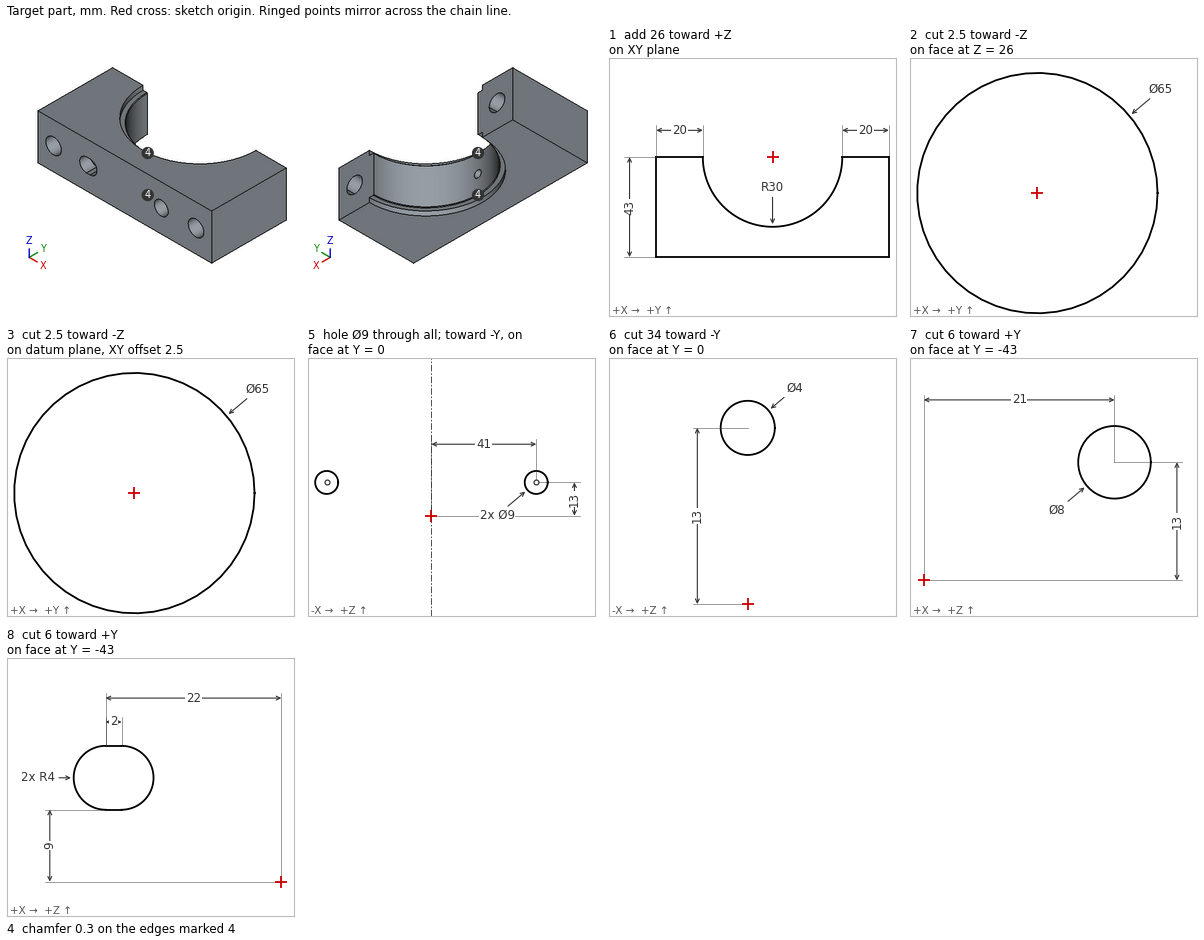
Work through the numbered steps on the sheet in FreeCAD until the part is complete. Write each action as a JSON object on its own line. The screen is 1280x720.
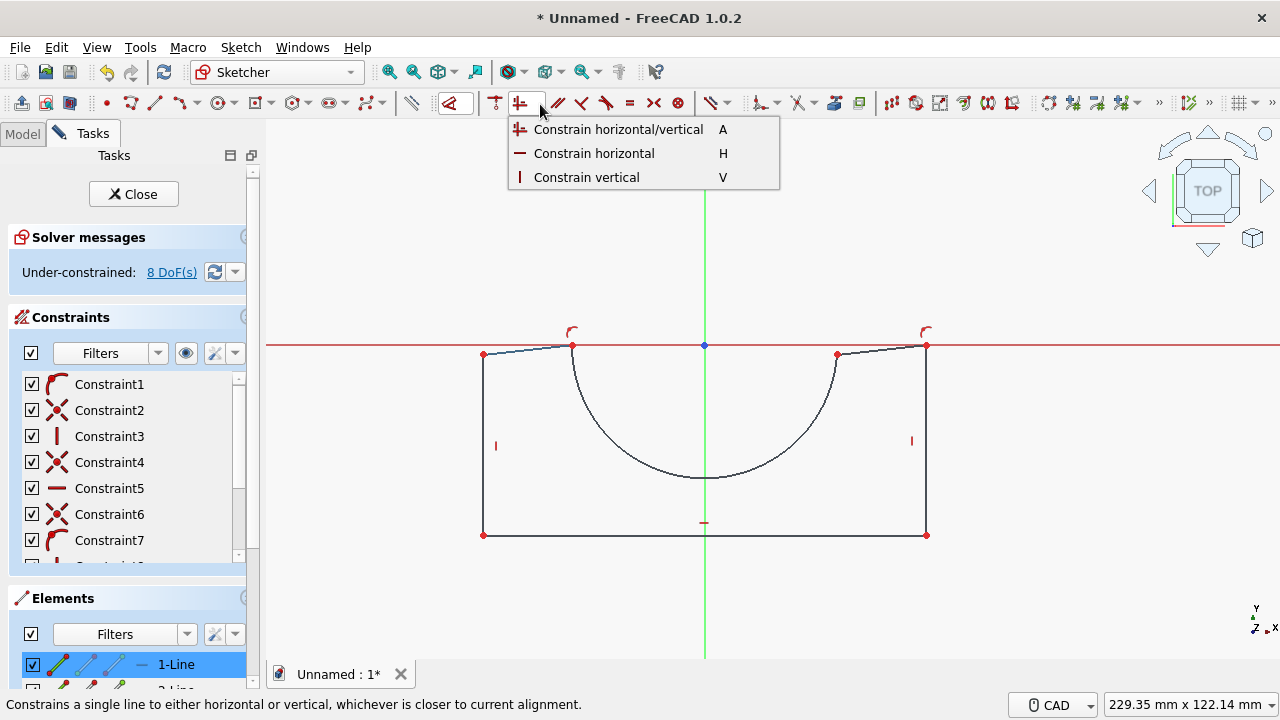
{"action": "left_click", "coordinate": [644, 153]}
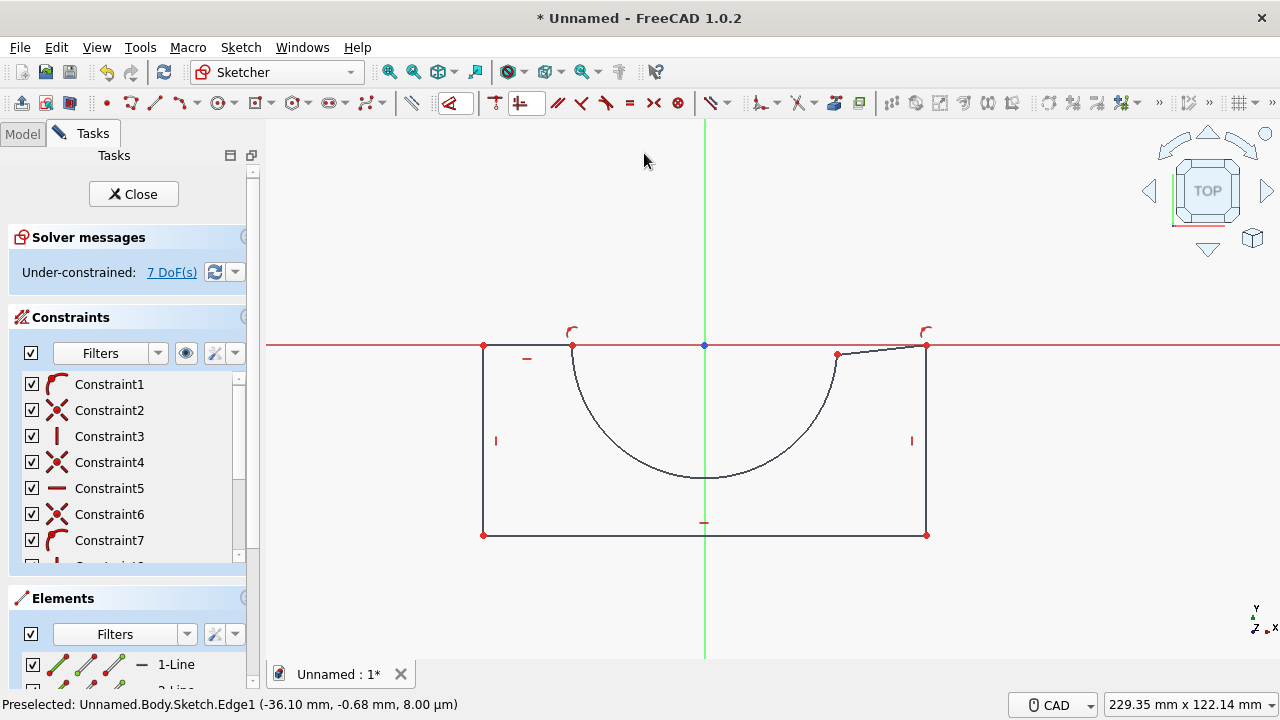
{"action": "left_click", "coordinate": [899, 348]}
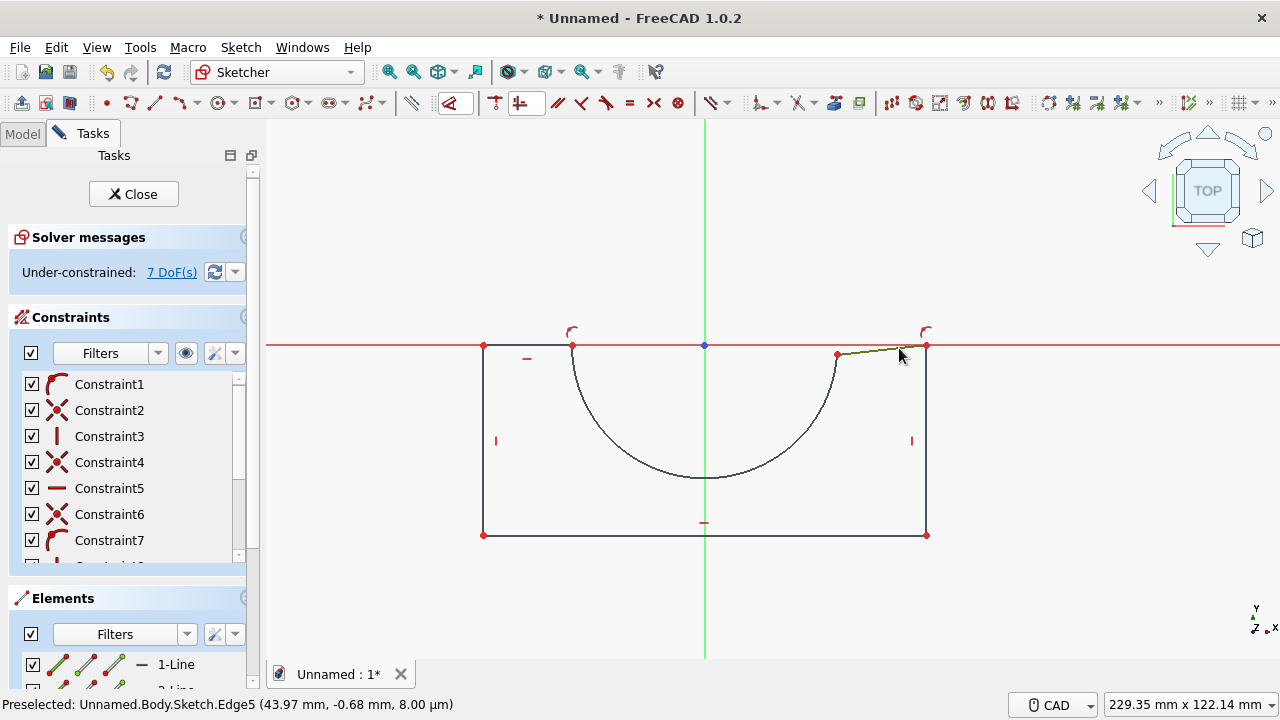
{"action": "key", "text": "h"}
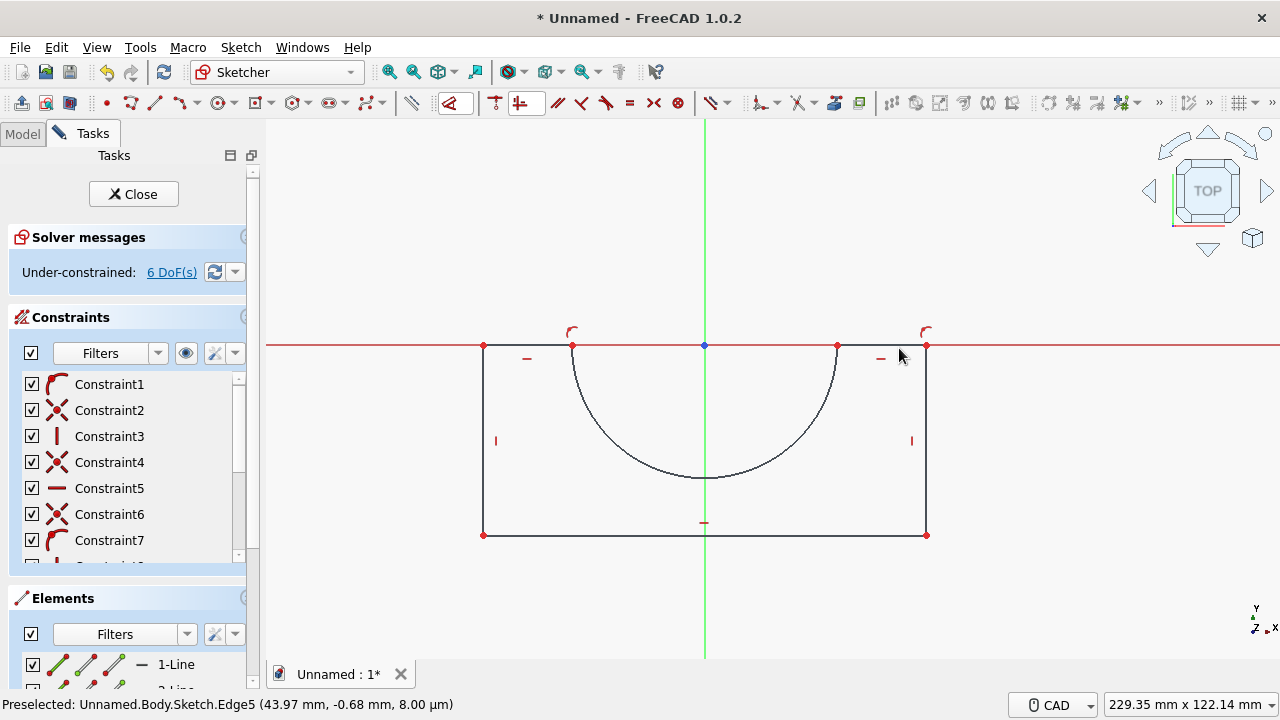
{"action": "left_click_drag", "start_coordinate": [695, 335], "coordinate": [715, 356]}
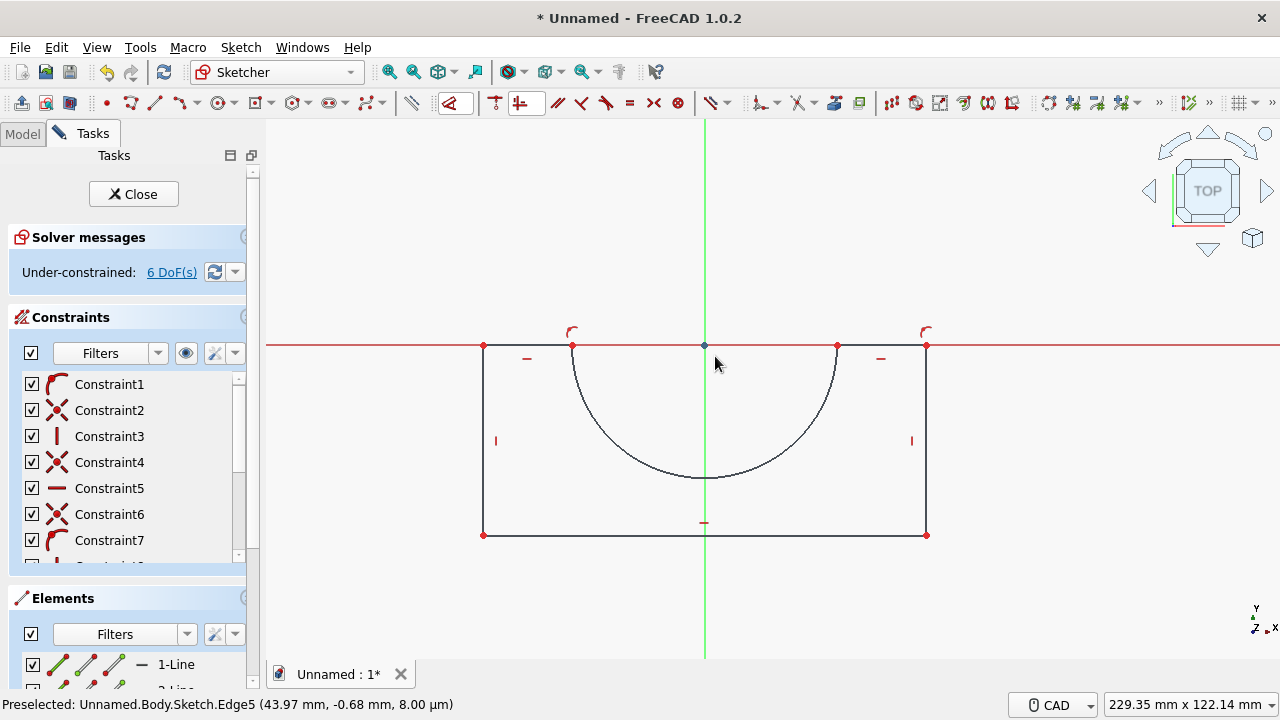
{"action": "left_click", "coordinate": [496, 104]}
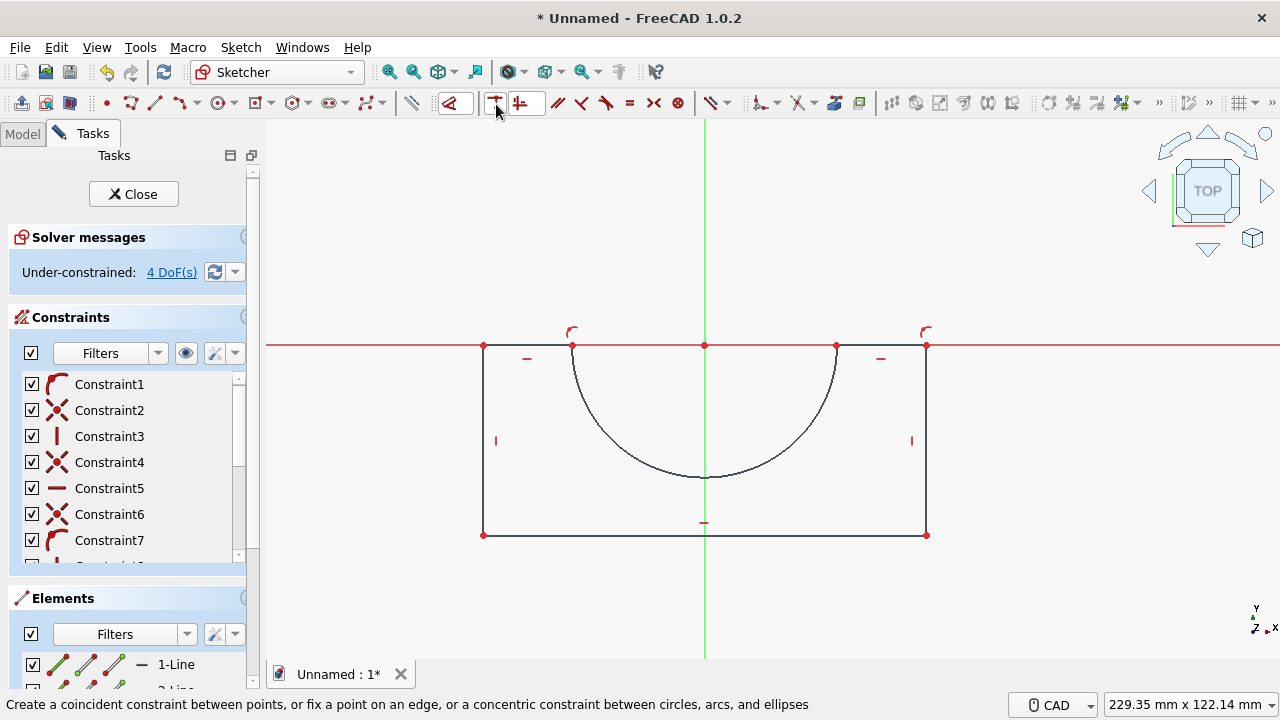
{"action": "left_click", "coordinate": [627, 452]}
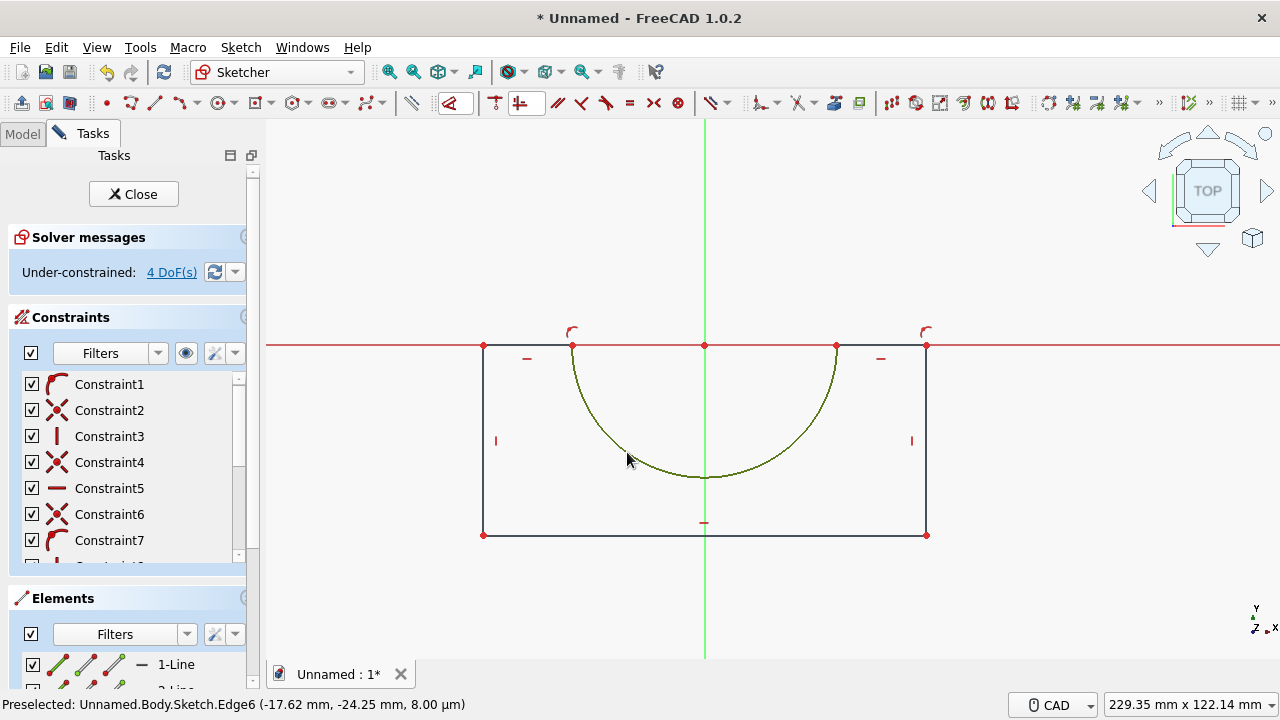
{"action": "left_click", "coordinate": [468, 104]}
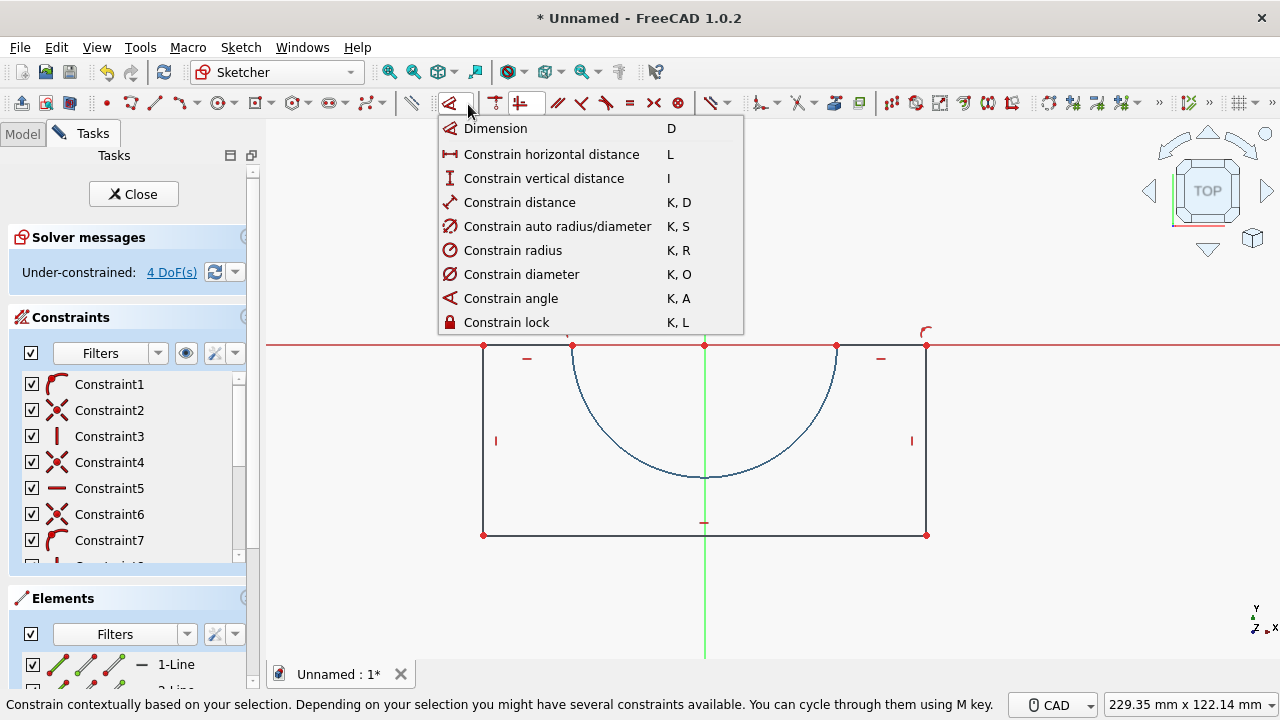
{"action": "left_click", "coordinate": [591, 250]}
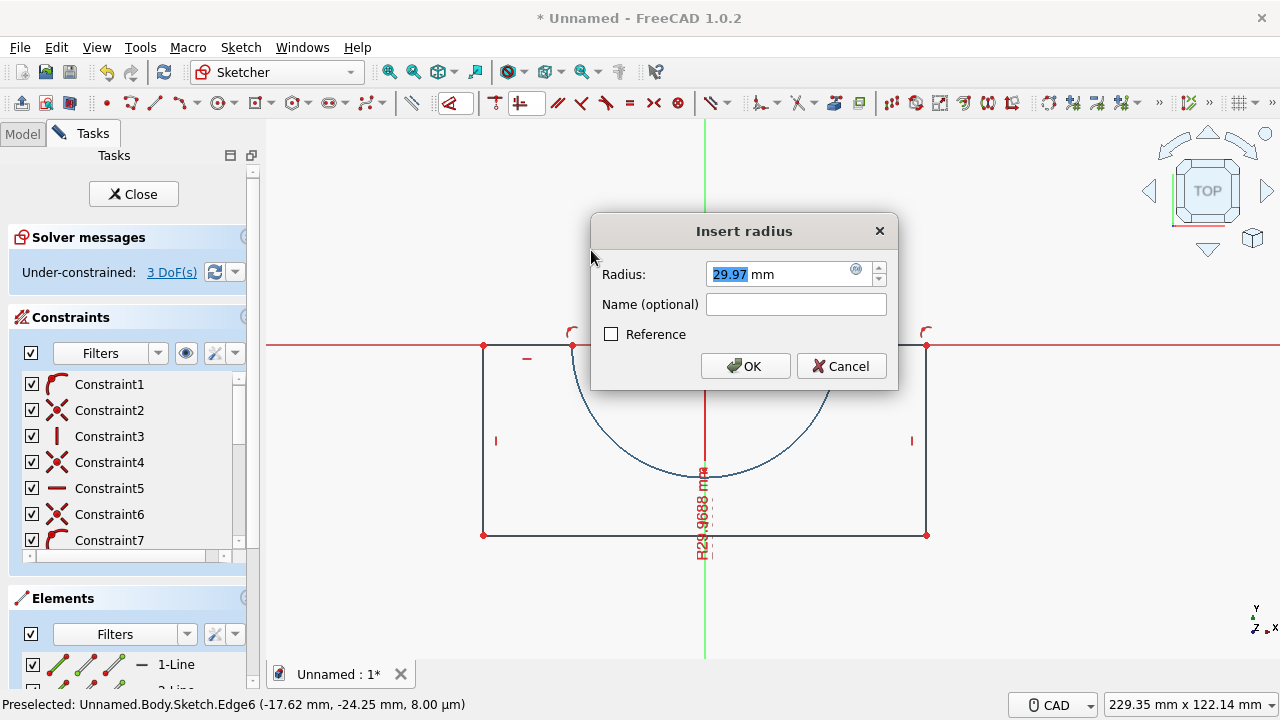
{"action": "type", "text": "30"}
{"action": "key", "text": "Return"}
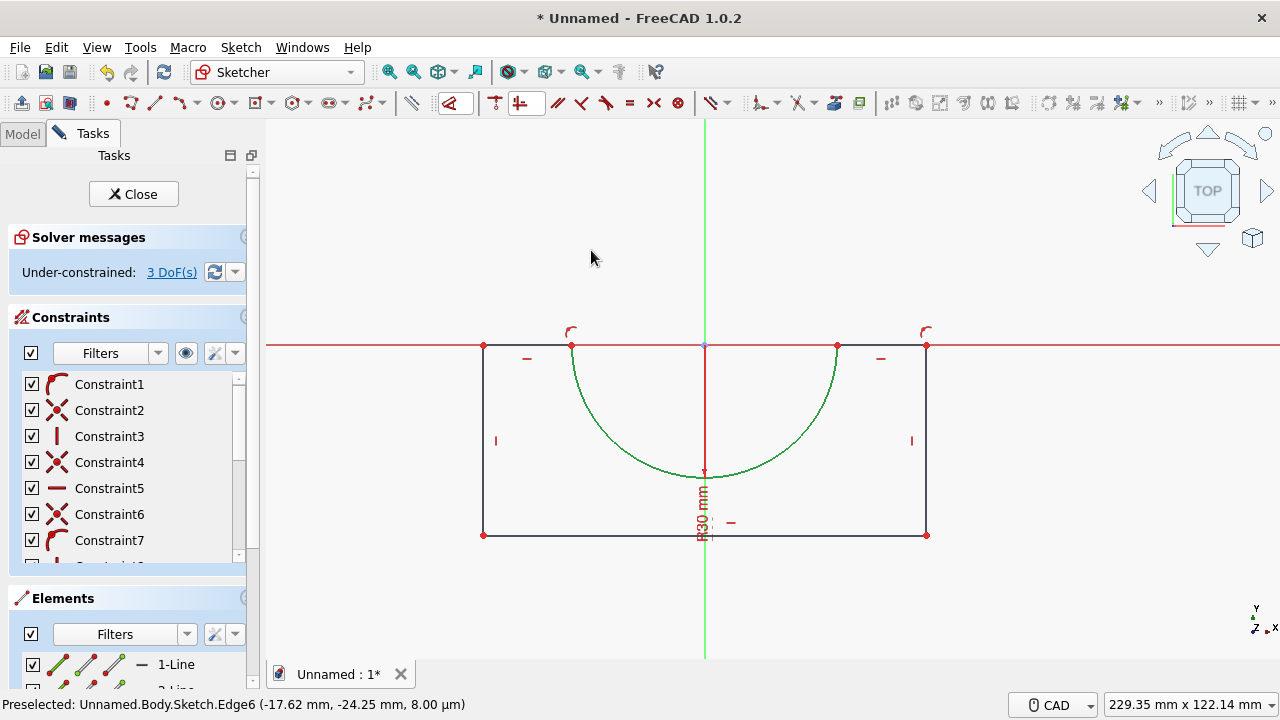
{"action": "left_click", "coordinate": [545, 345]}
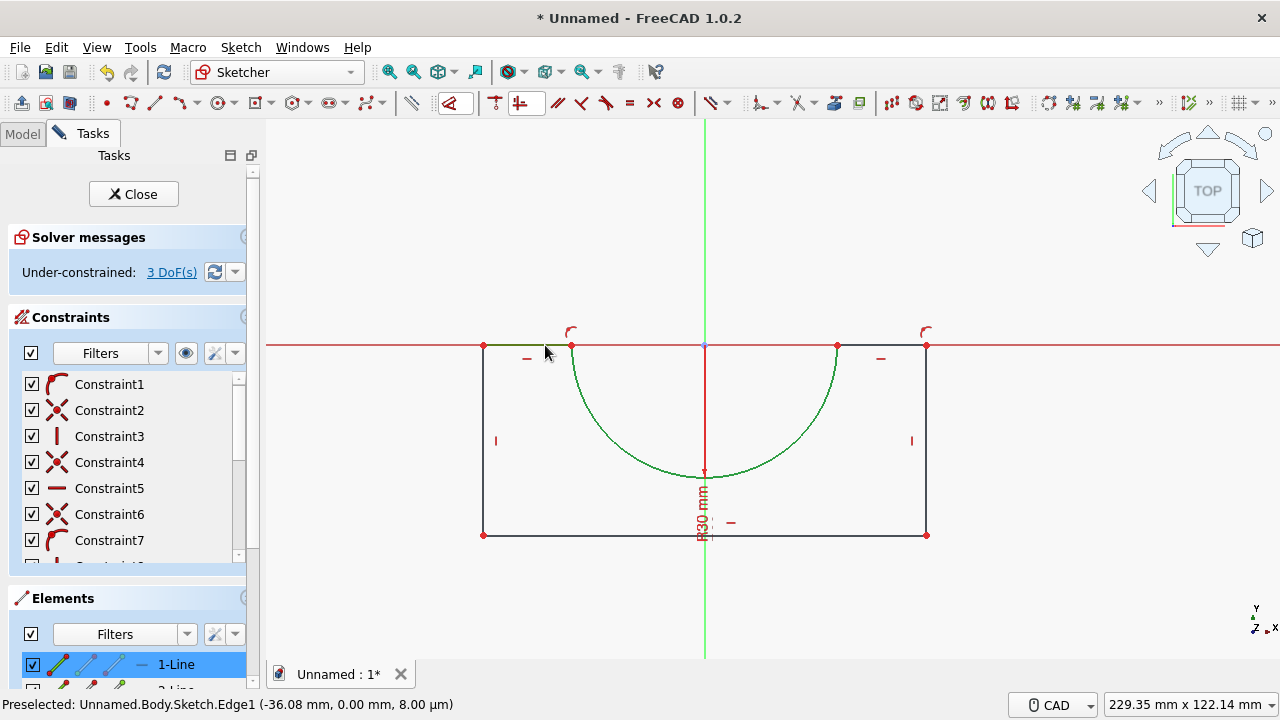
{"action": "key", "text": "l"}